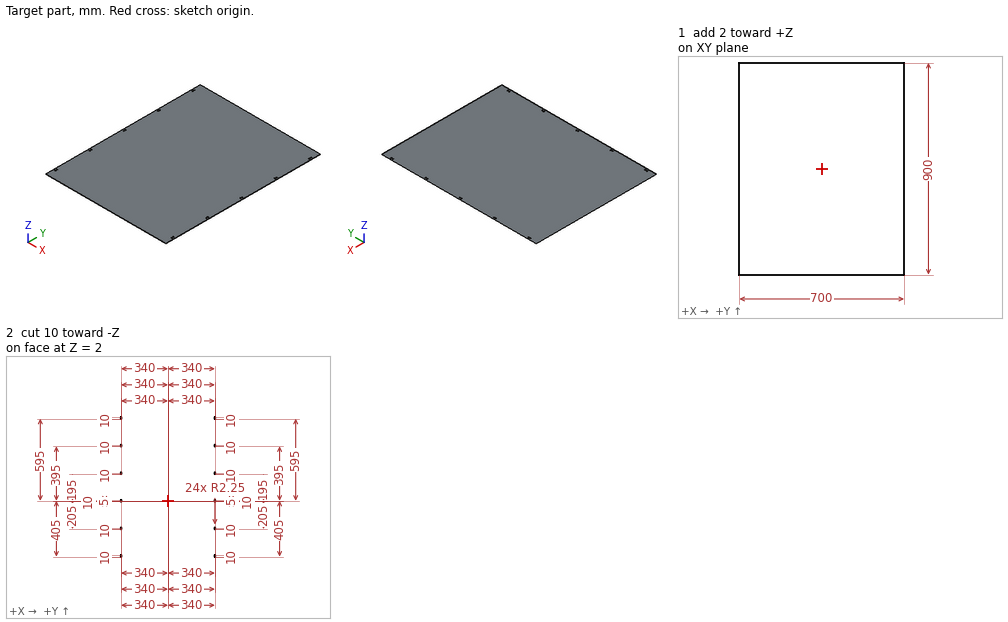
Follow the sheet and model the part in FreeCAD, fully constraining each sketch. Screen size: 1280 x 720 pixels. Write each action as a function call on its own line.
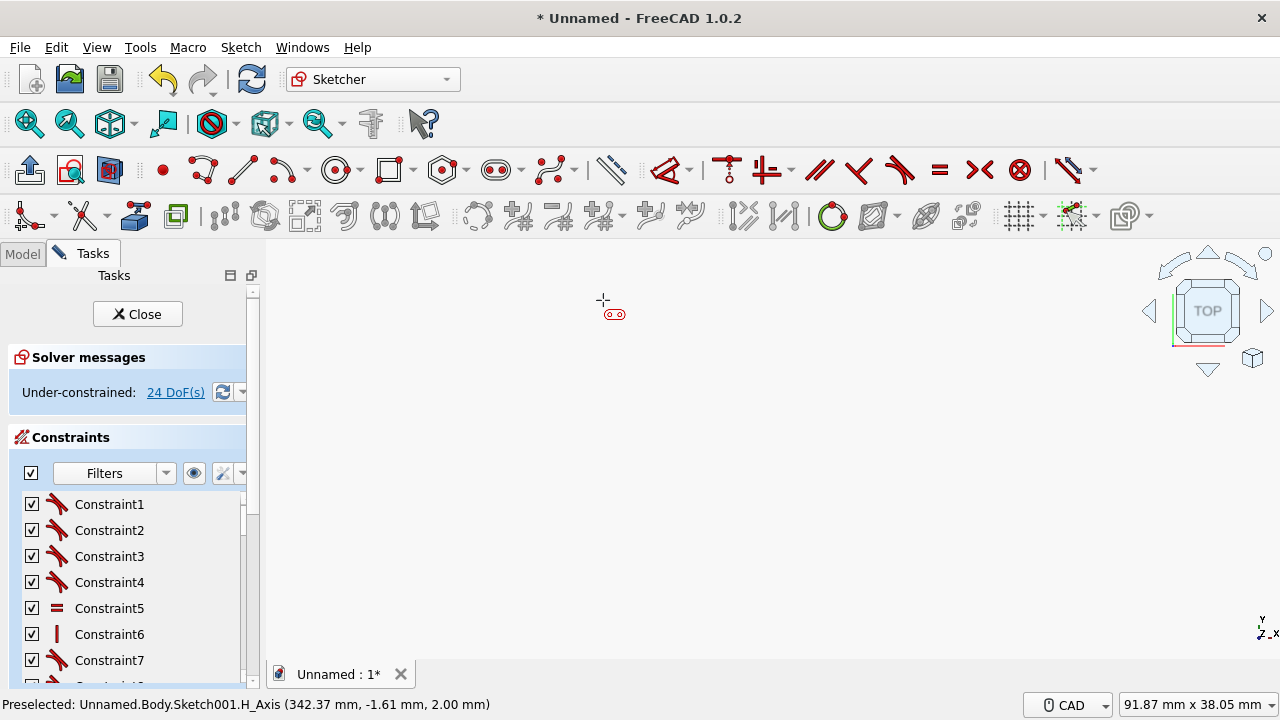
scroll(603, 300, down, 18)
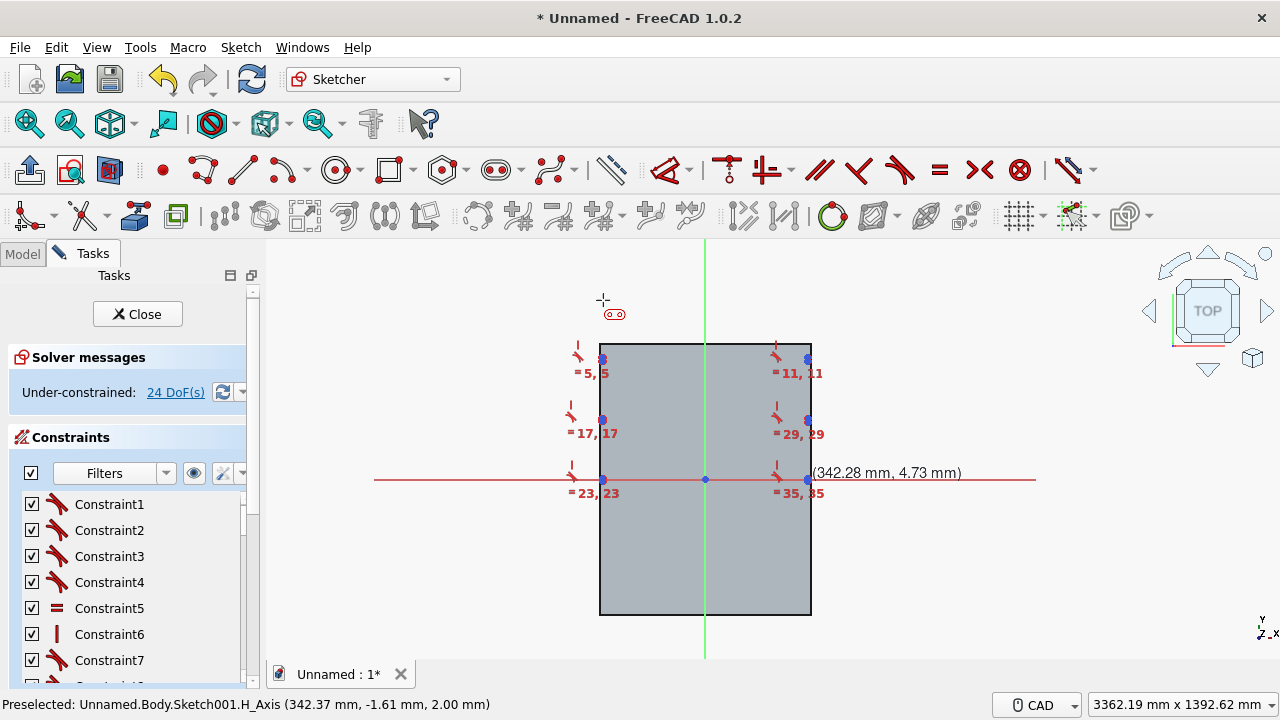
click(603, 300)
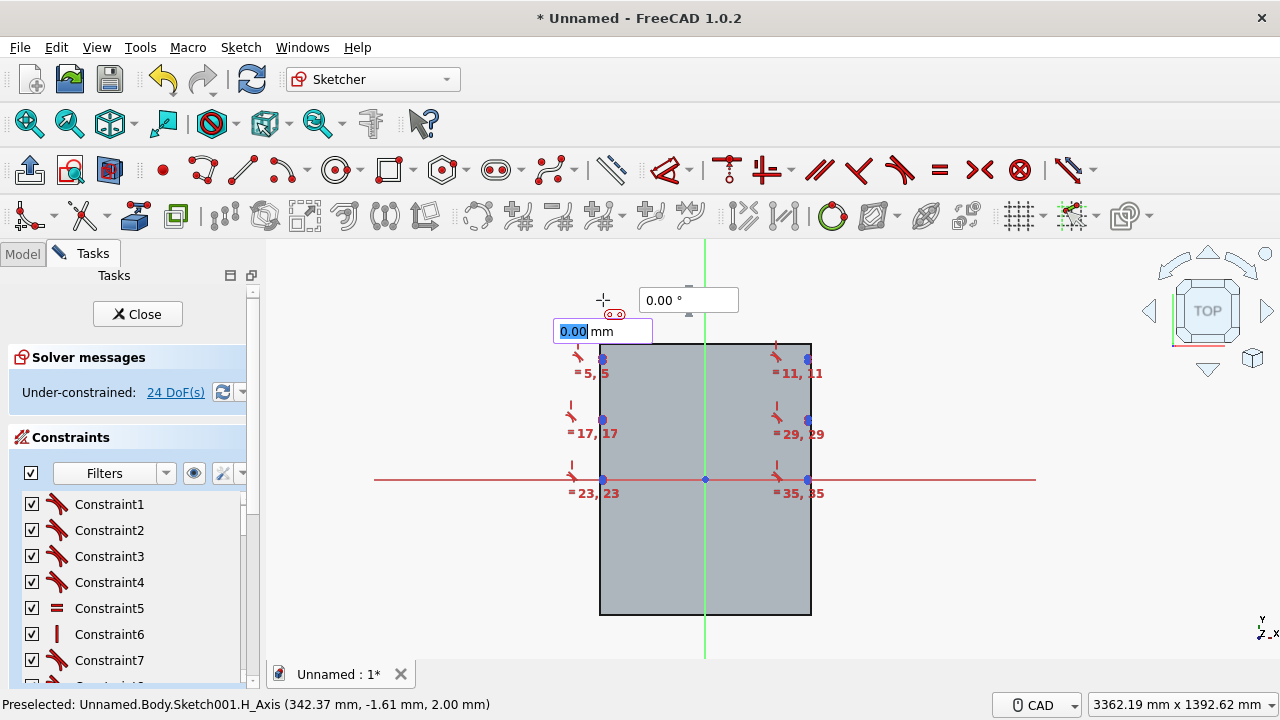
scroll(603, 297, up, 9)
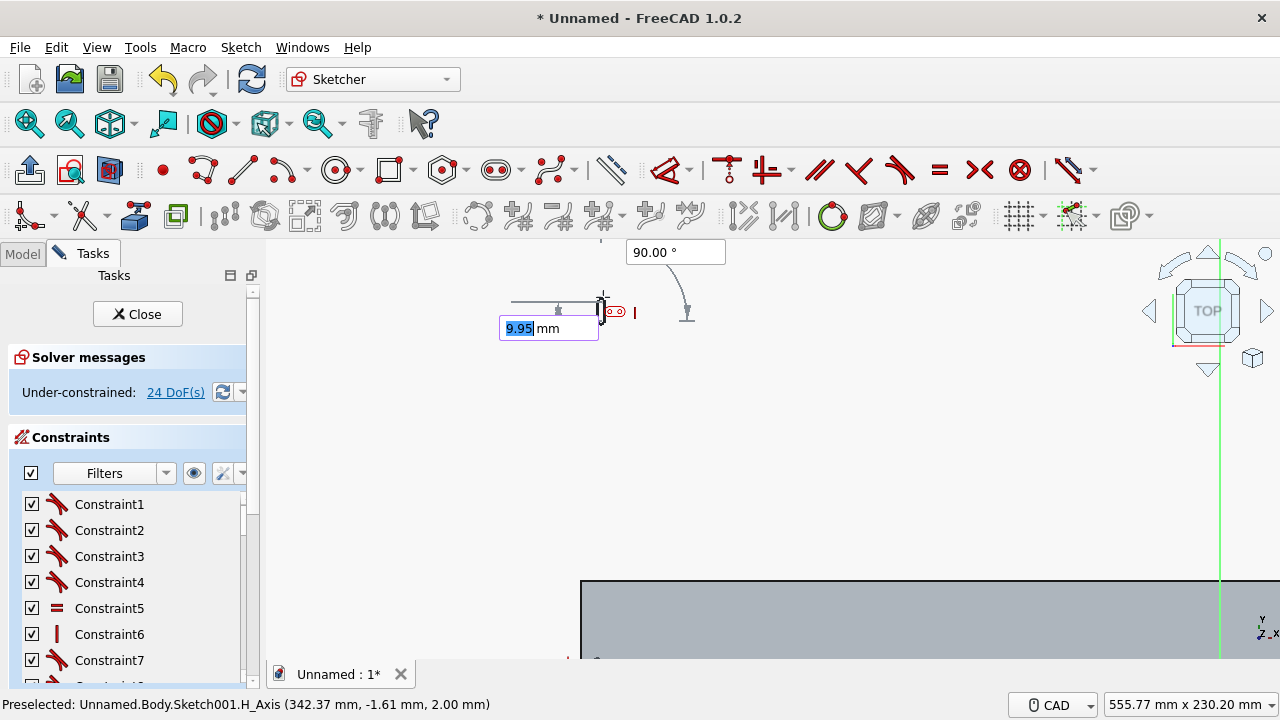
click(601, 298)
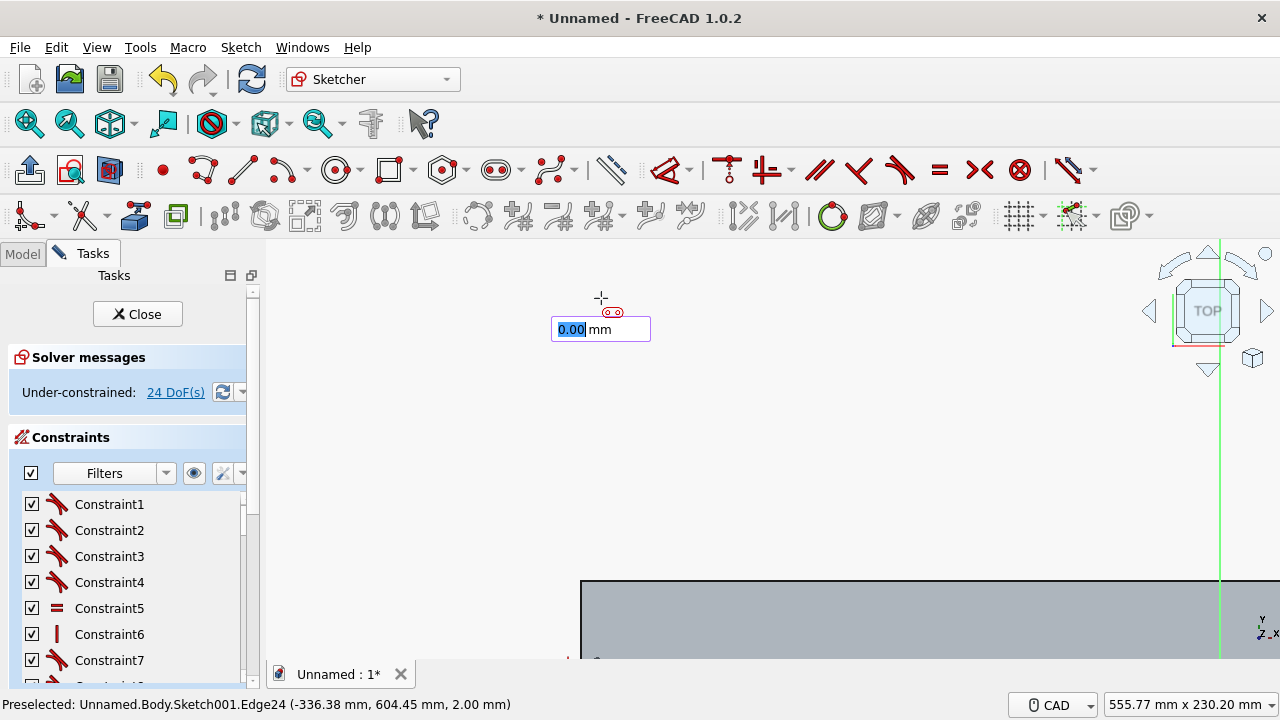
scroll(595, 307, up, 7)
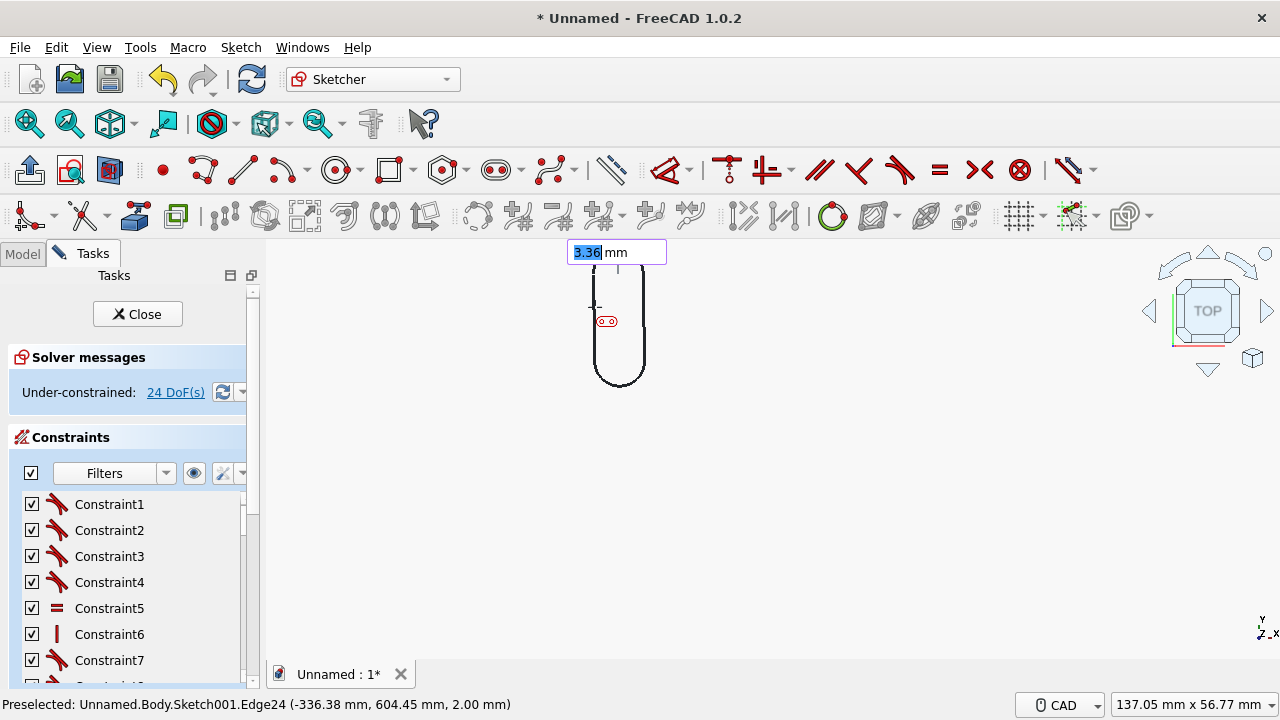
click(595, 306)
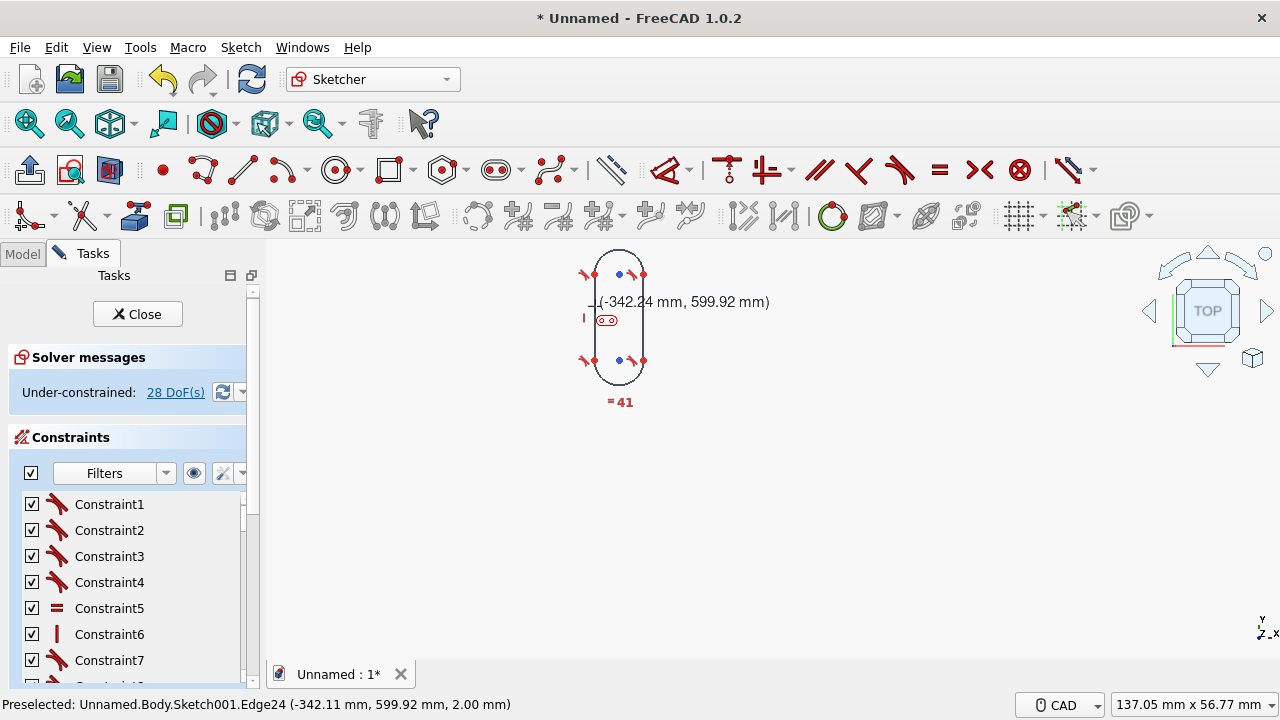
scroll(602, 298, down, 16)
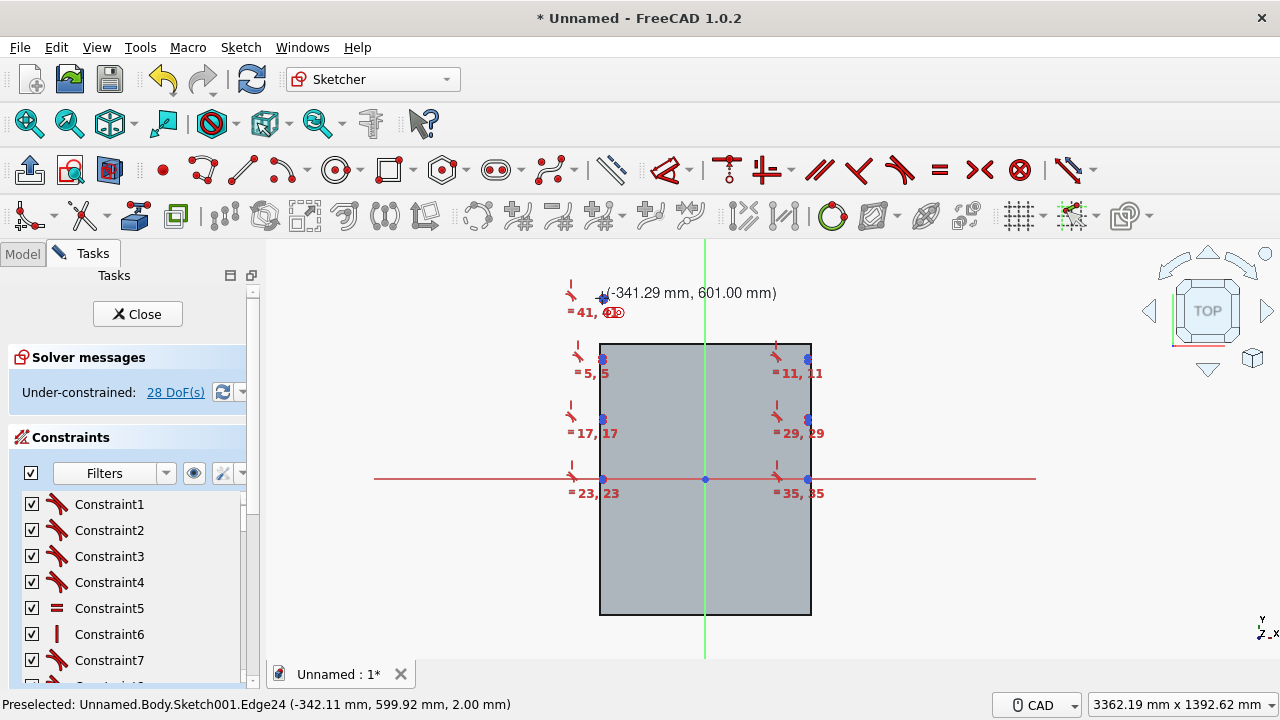
scroll(808, 300, up, 18)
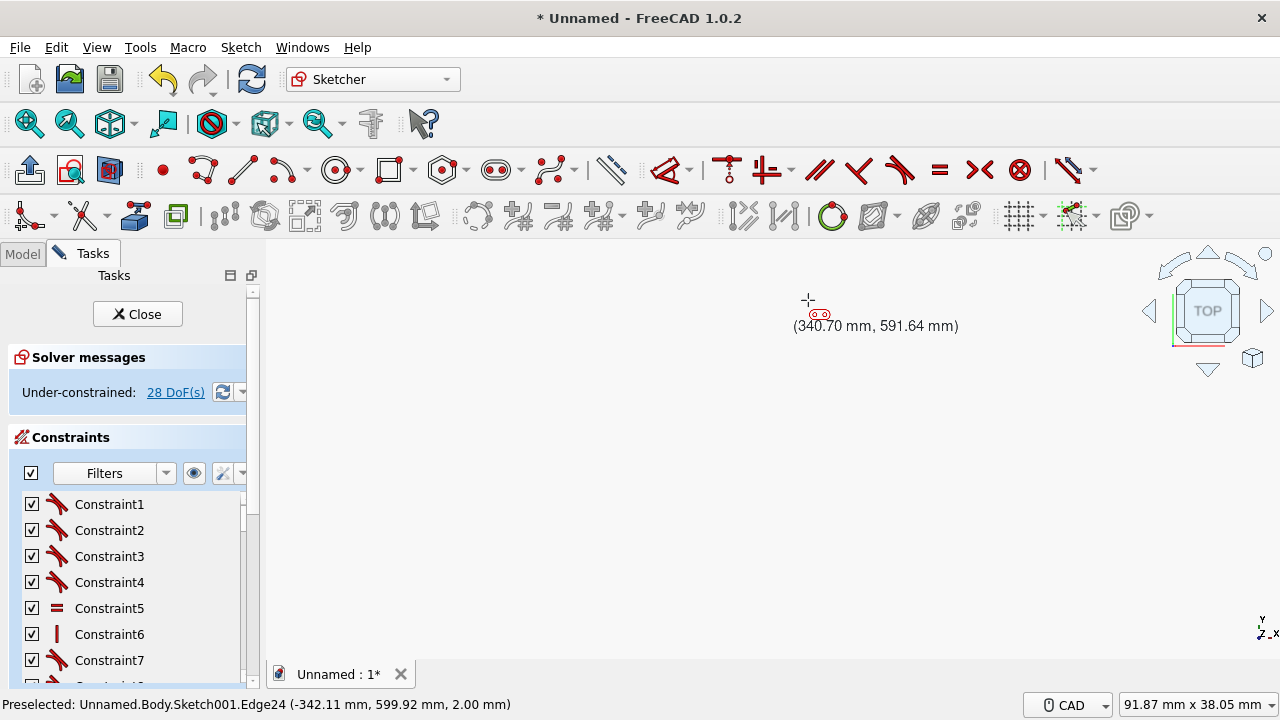
scroll(808, 300, down, 18)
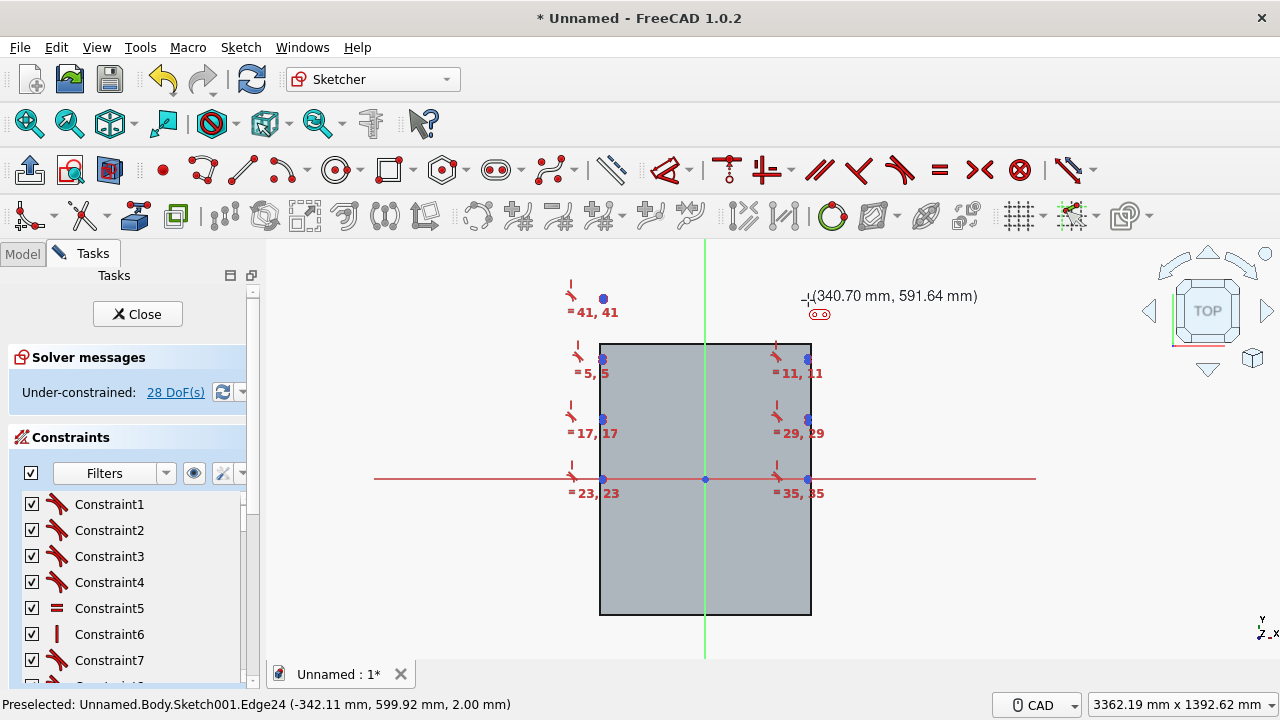
click(808, 300)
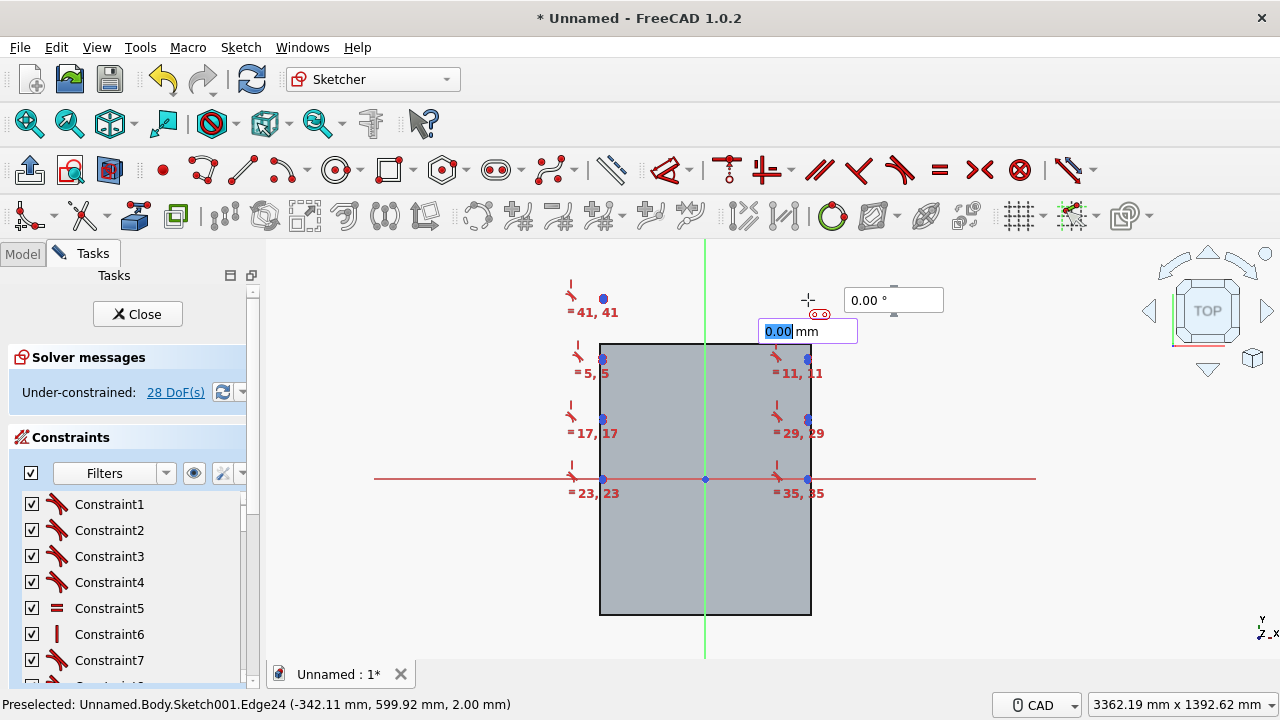
scroll(808, 297, up, 9)